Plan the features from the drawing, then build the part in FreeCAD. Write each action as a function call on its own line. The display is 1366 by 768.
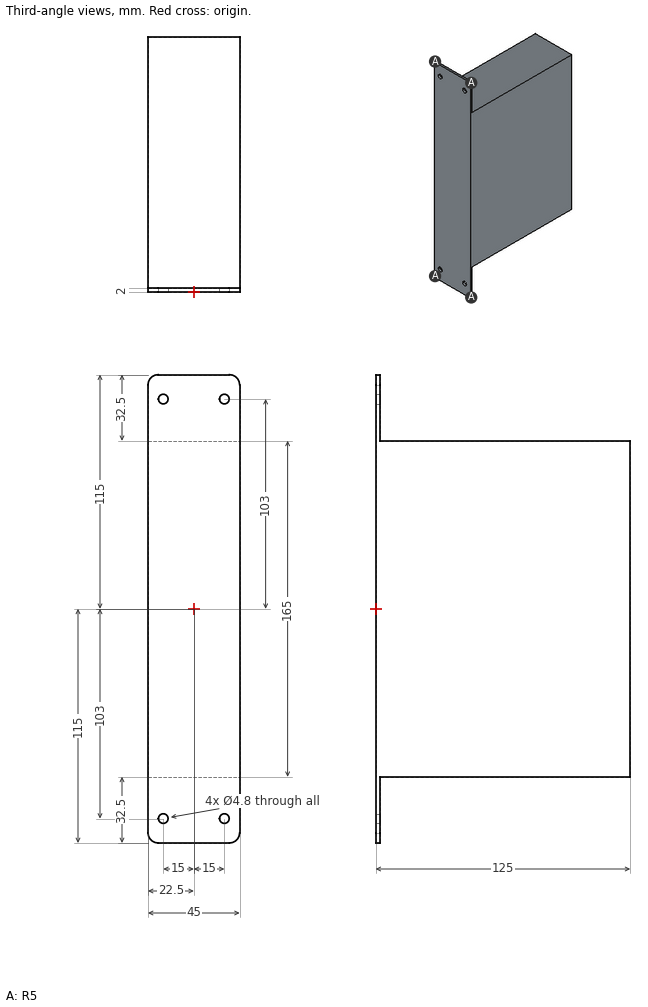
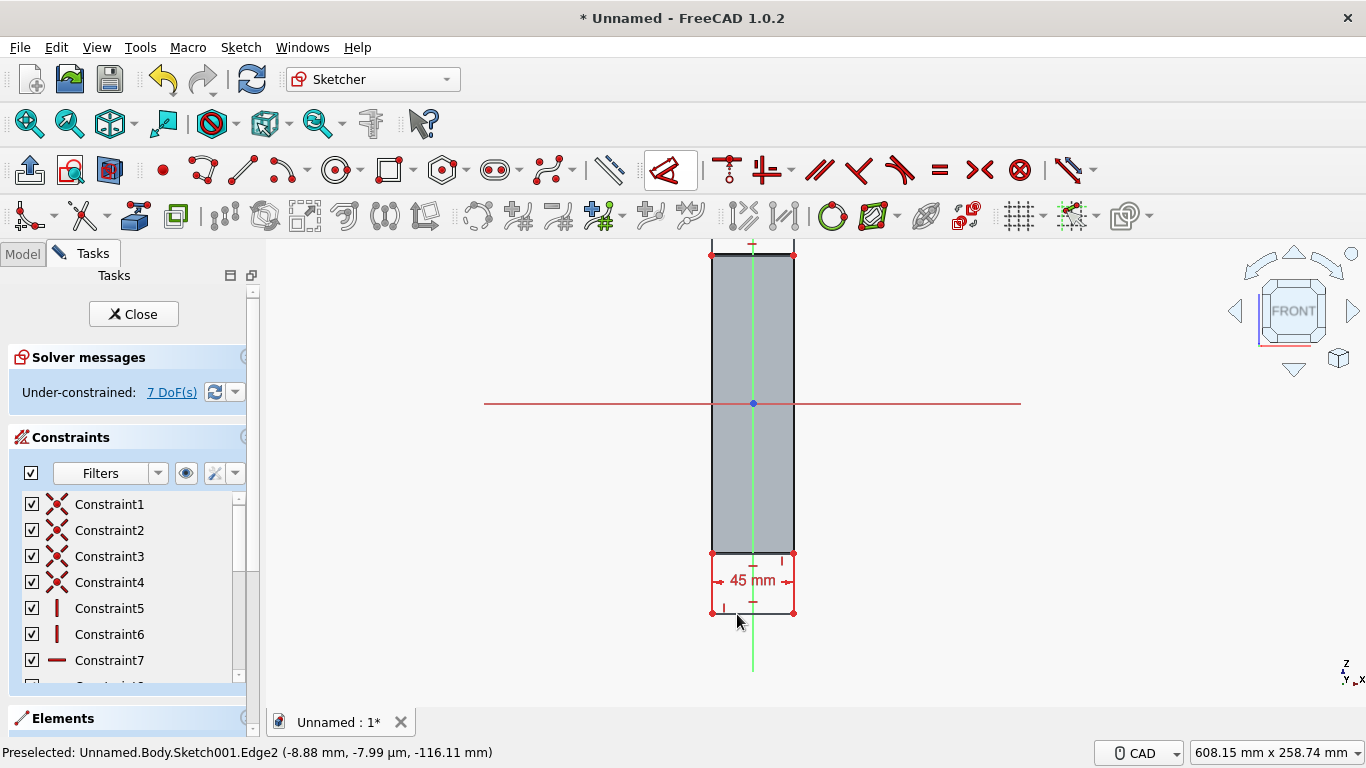
scroll(736, 614, down, 2)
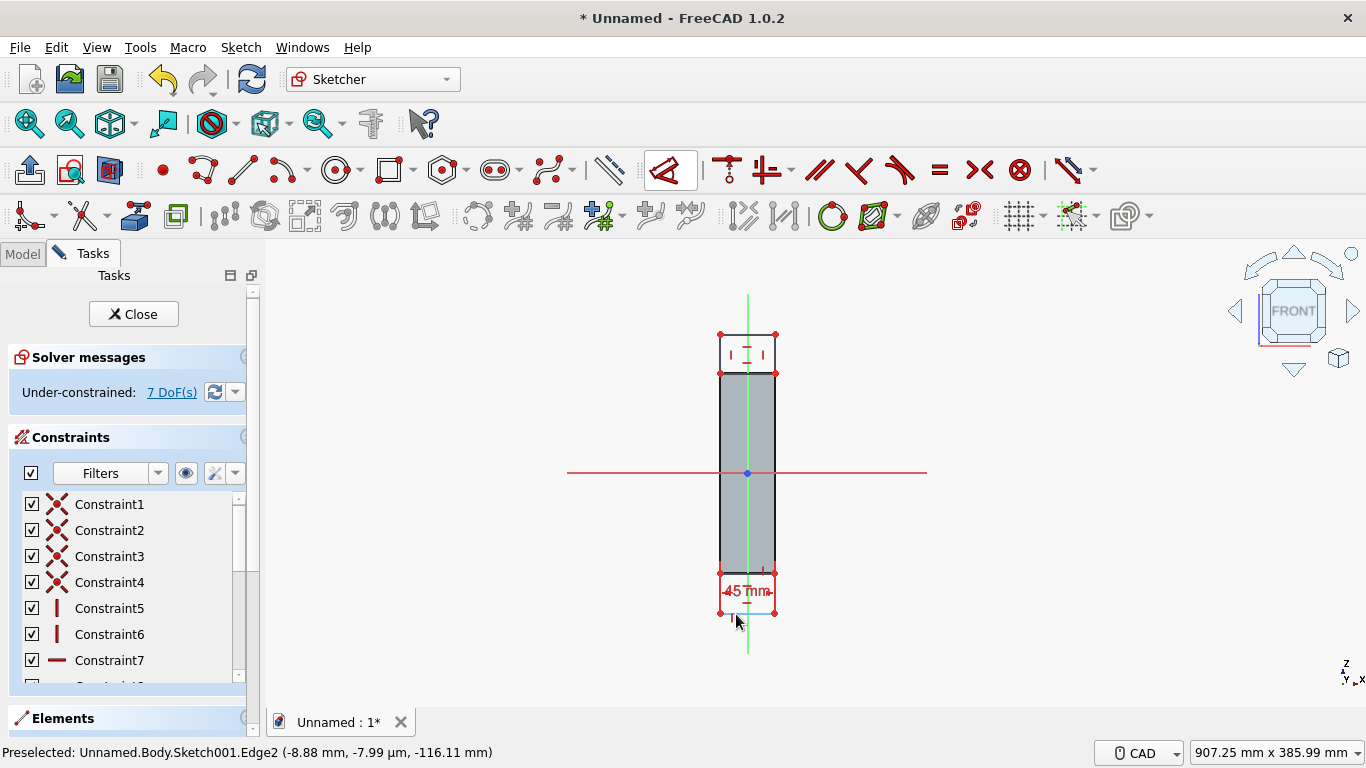
scroll(736, 374, up, 2)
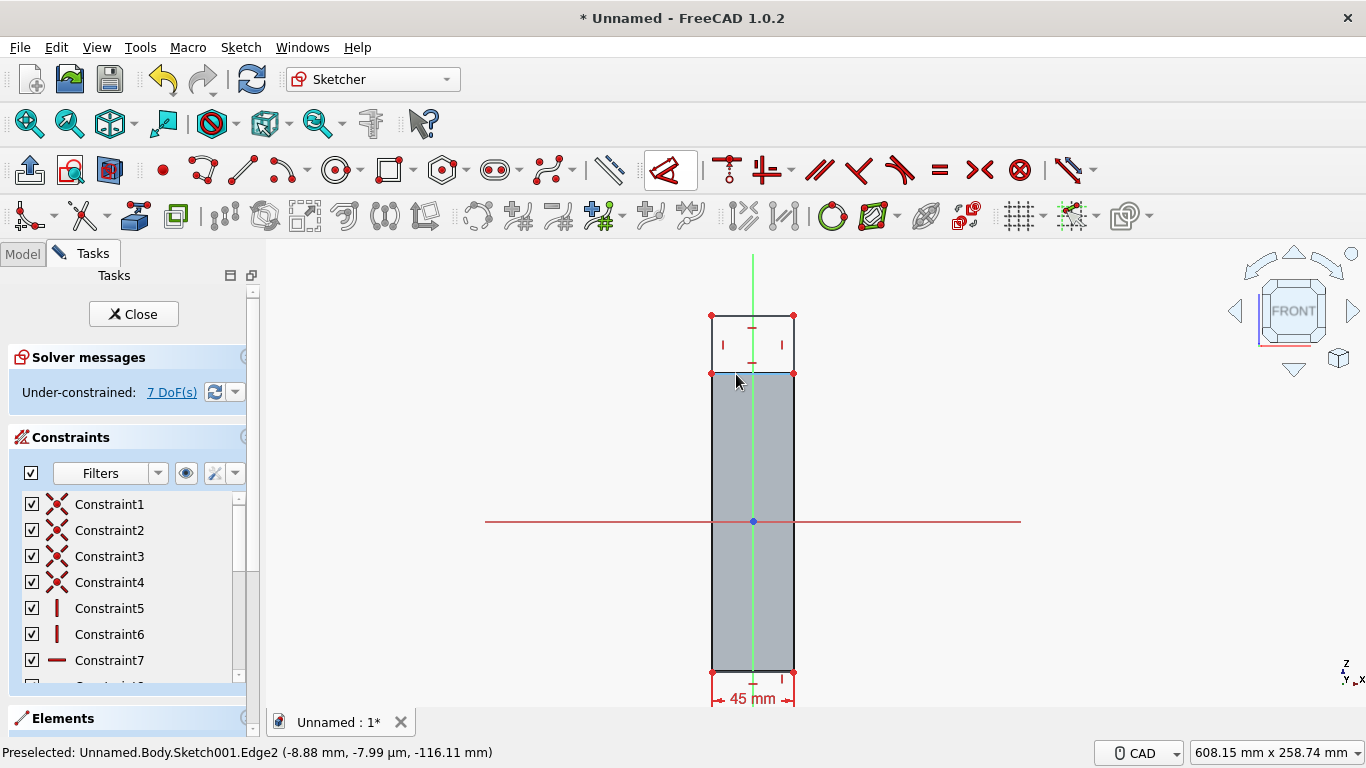
click(737, 374)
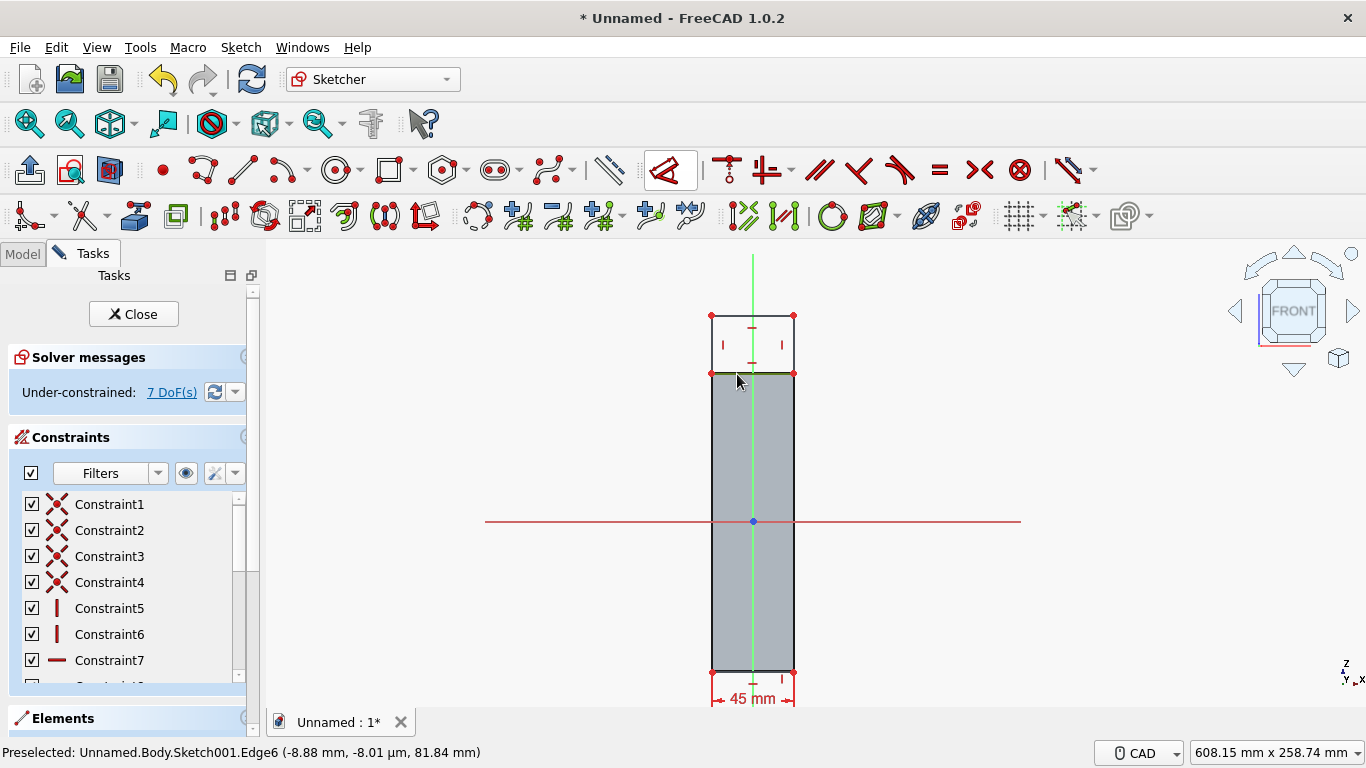
click(692, 170)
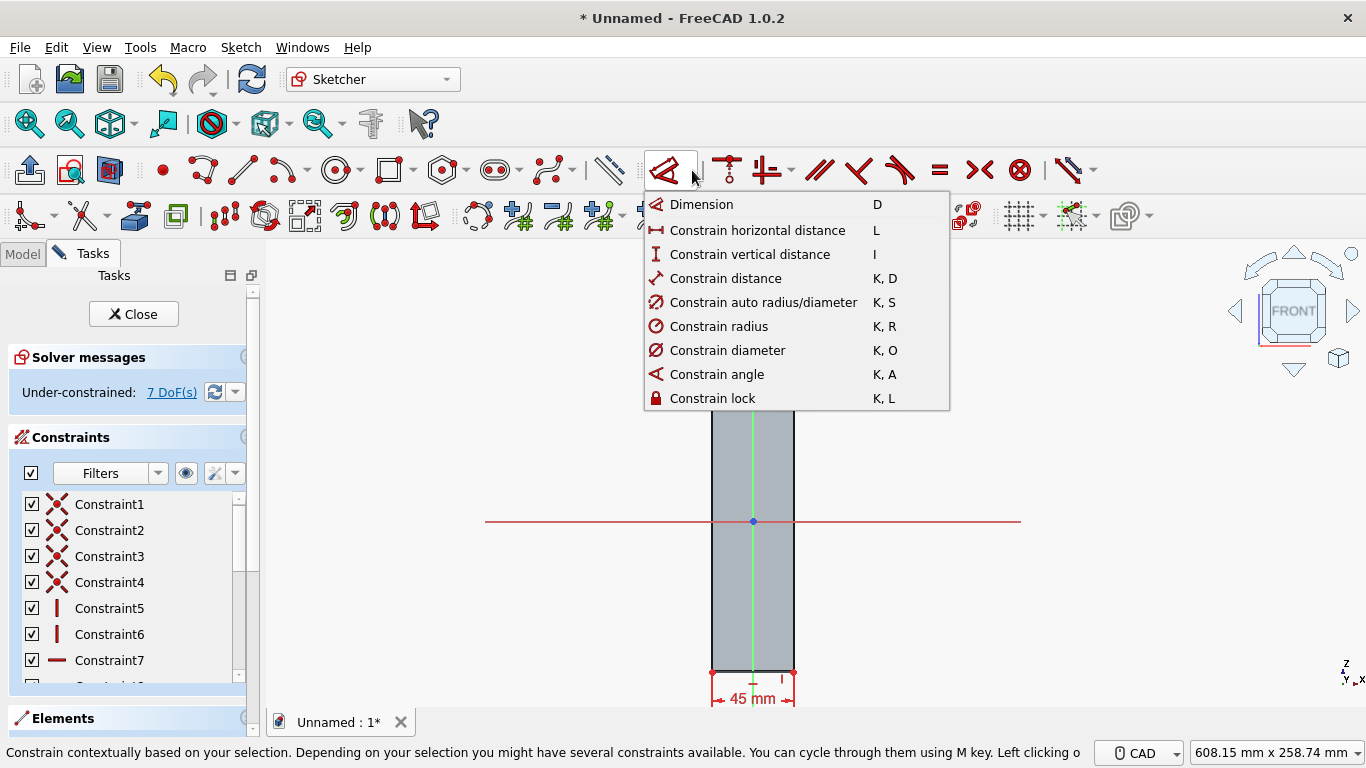
click(797, 230)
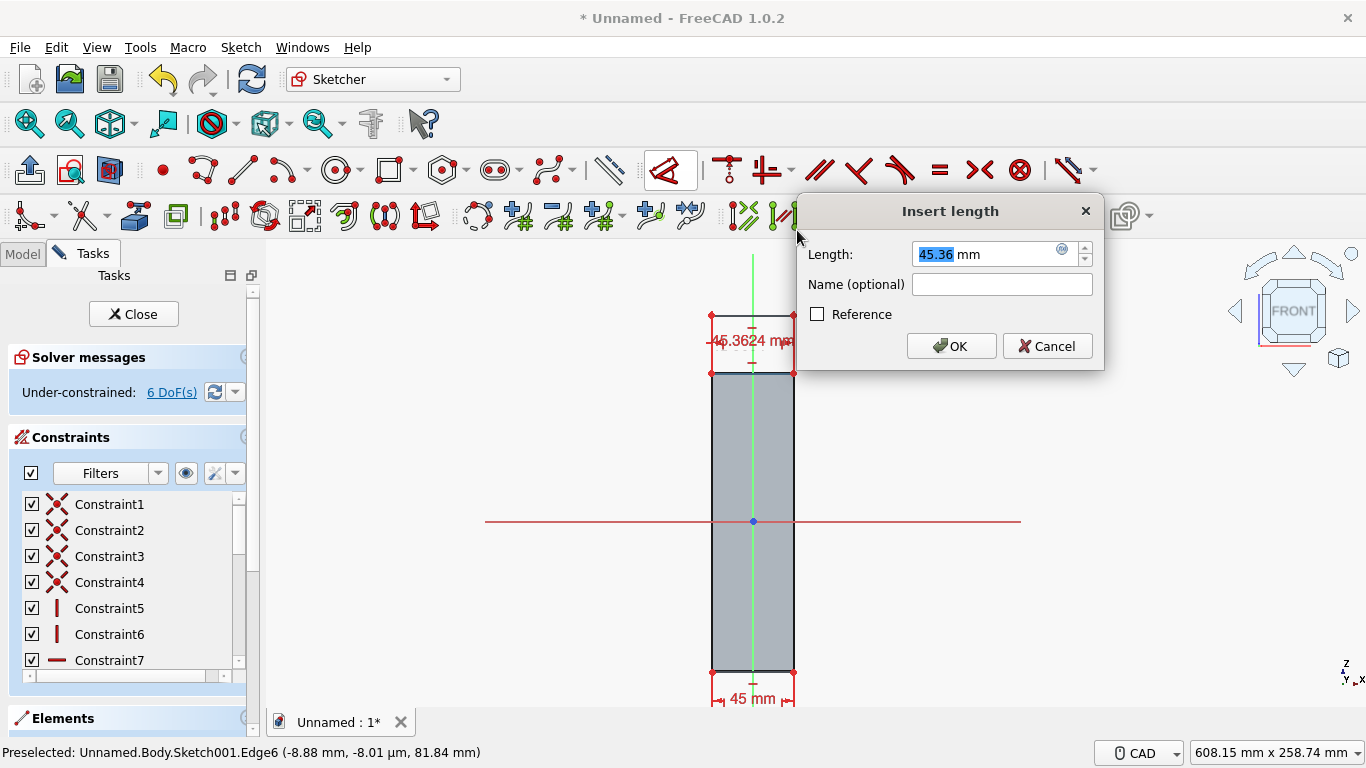
text(45)
key(Return)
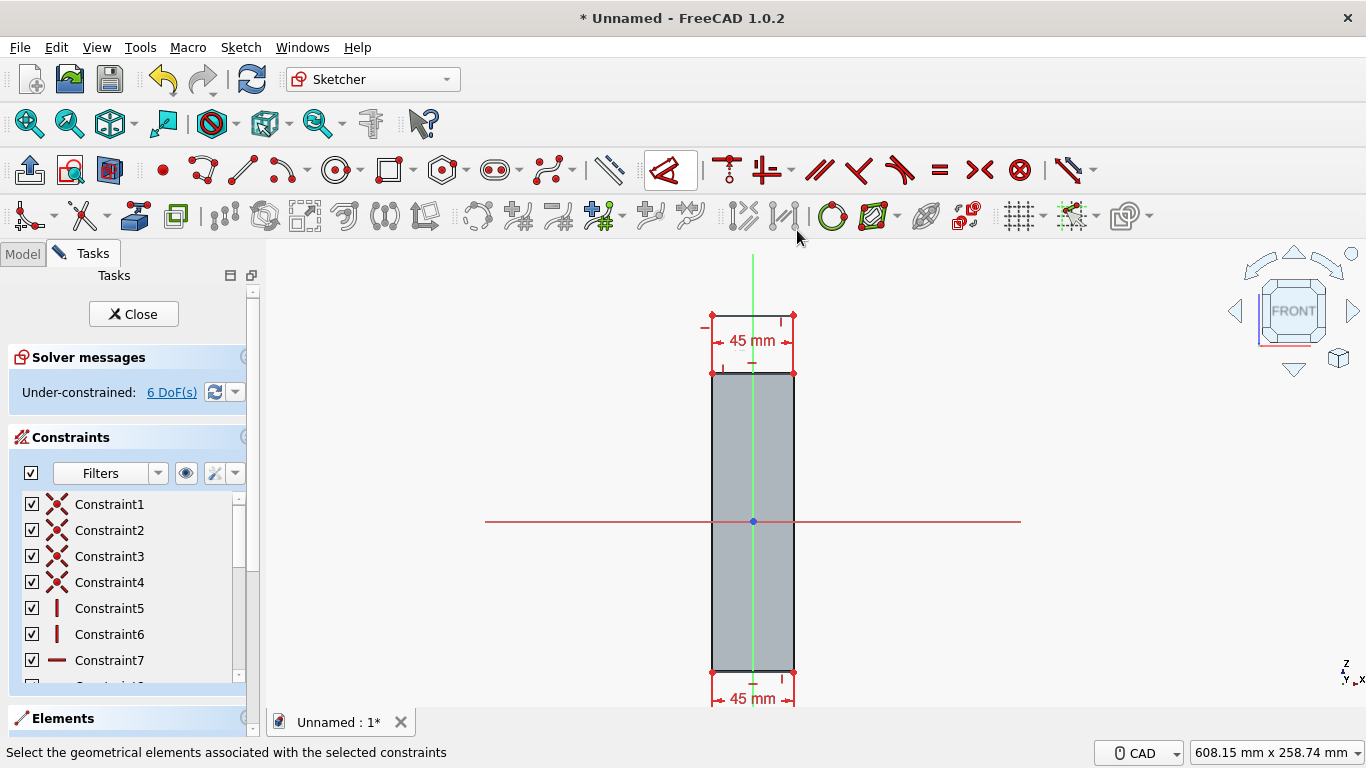
scroll(736, 374, down, 2)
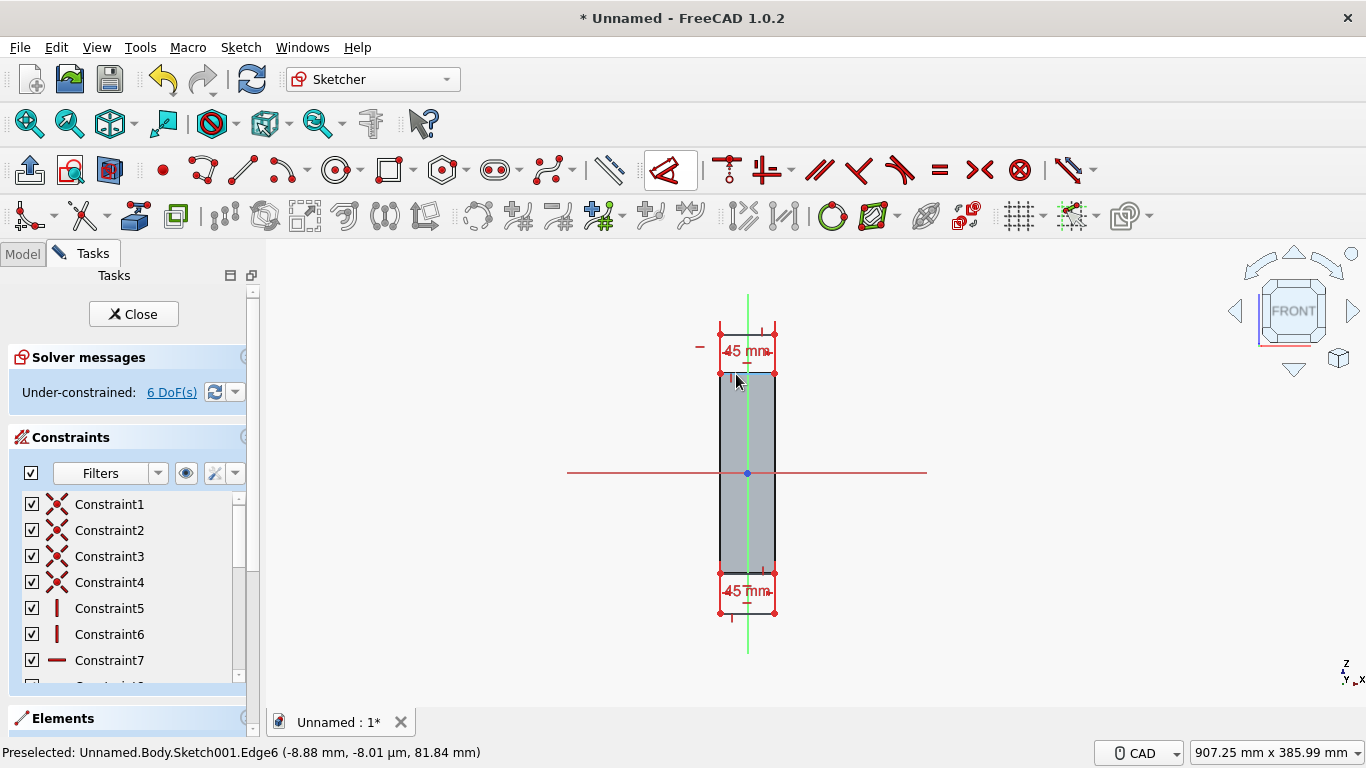
click(720, 586)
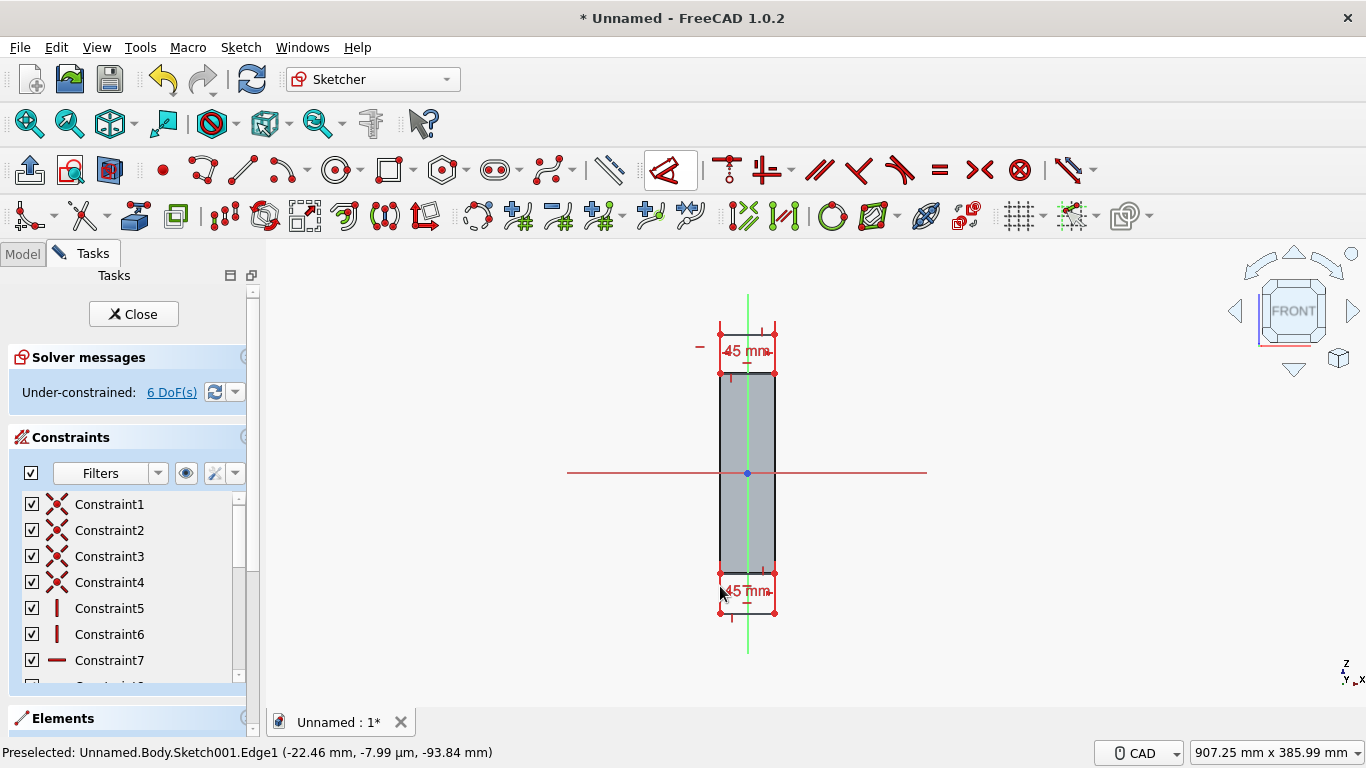
key(i)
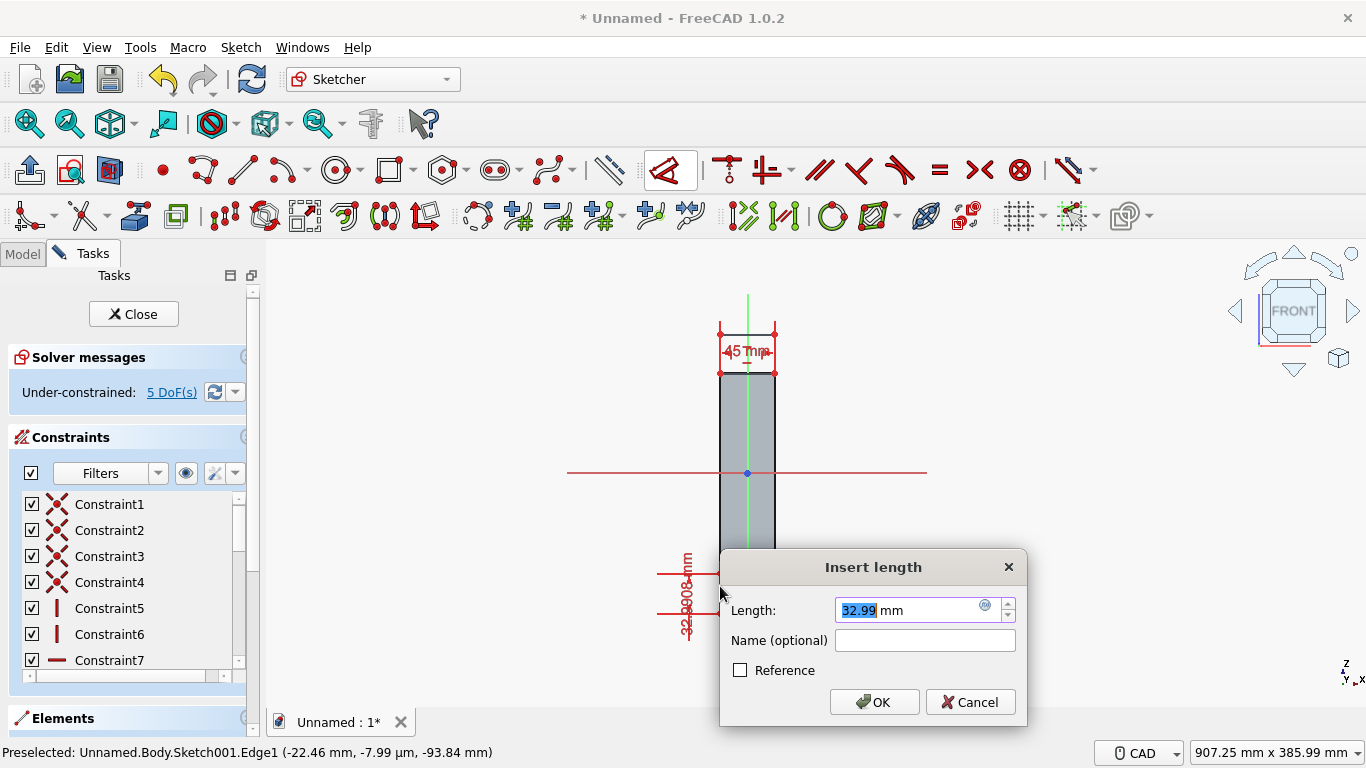
text(32.5)
key(Return)